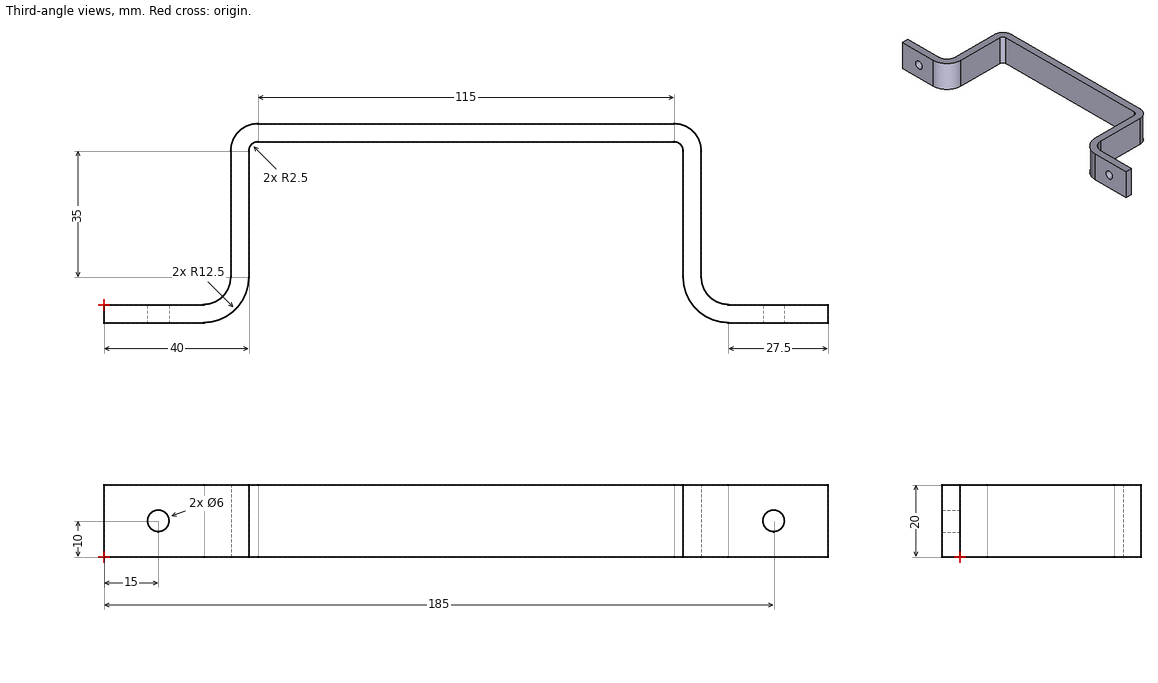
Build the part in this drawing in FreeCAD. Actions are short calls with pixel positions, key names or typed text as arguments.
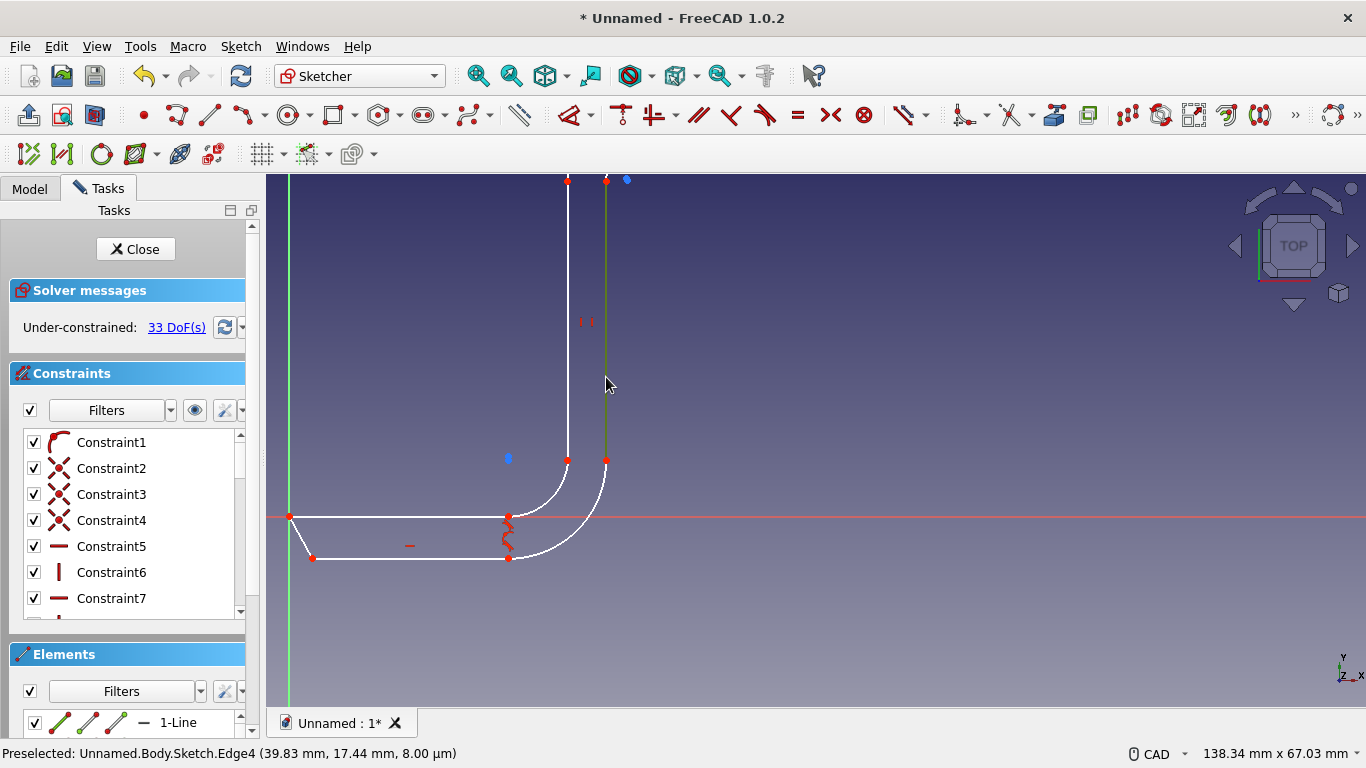
click(553, 548)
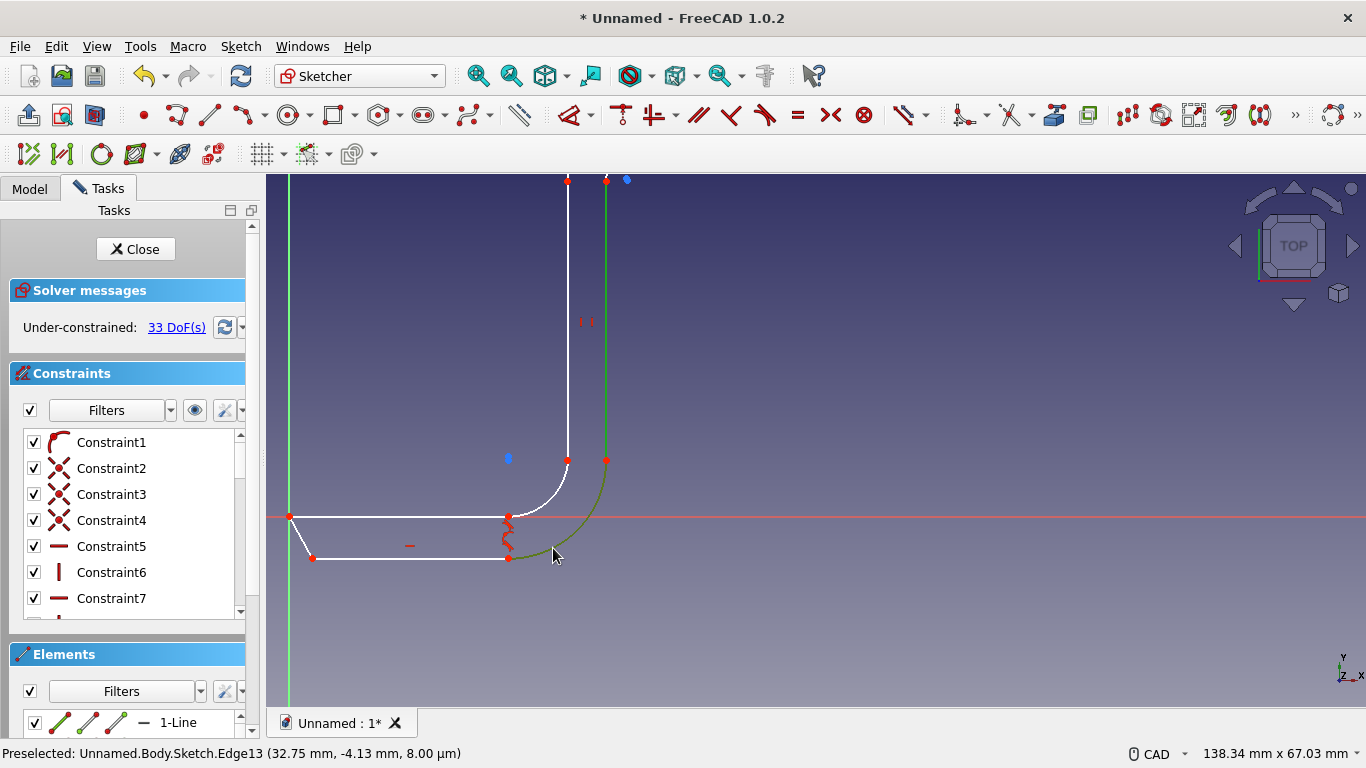
click(765, 116)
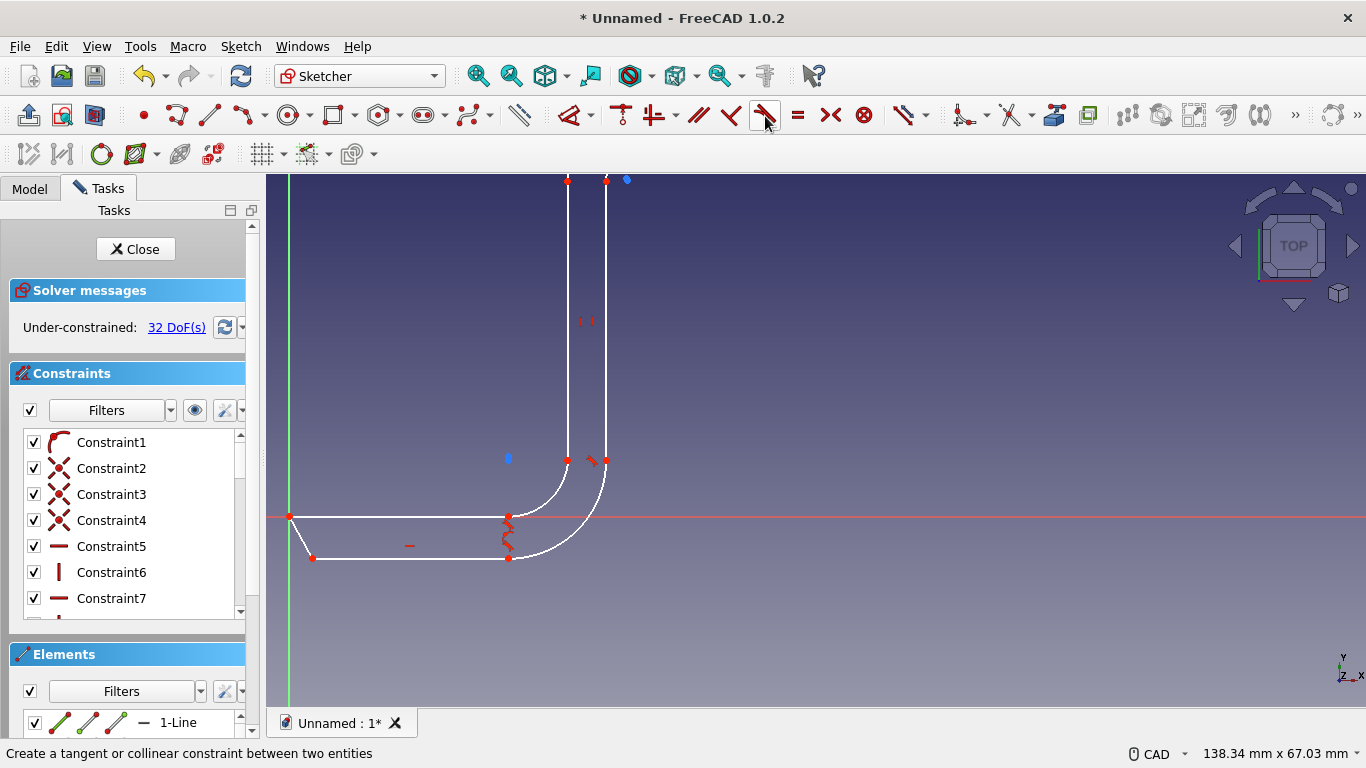
click(606, 377)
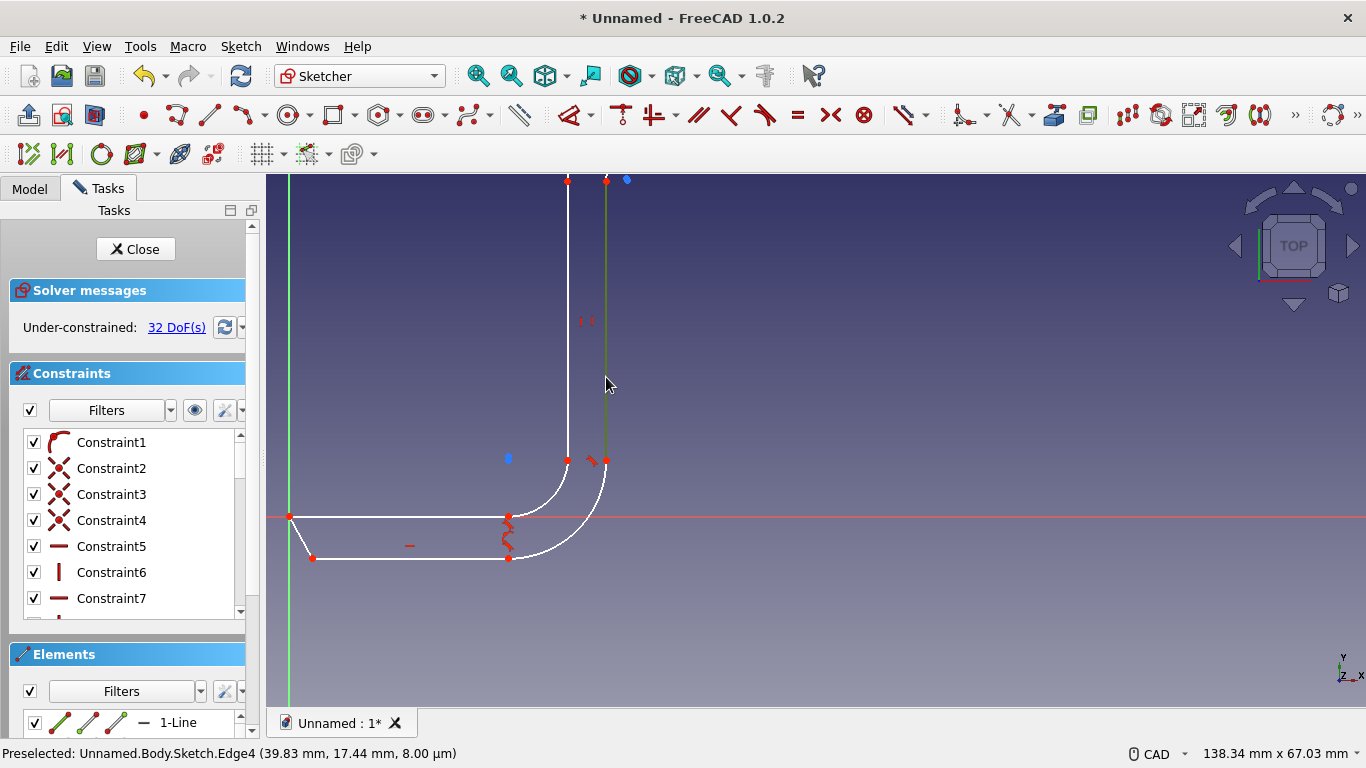
scroll(551, 500, down, 5)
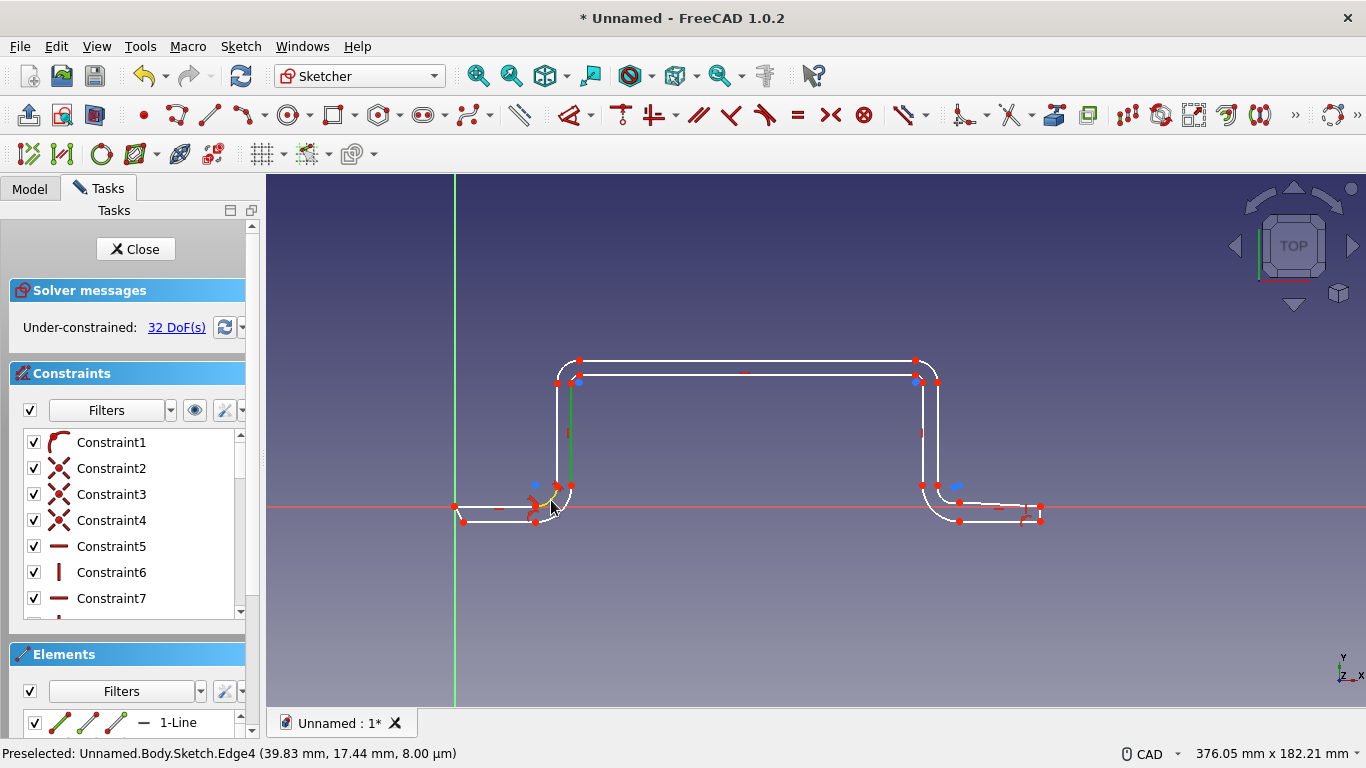
scroll(576, 376, up, 7)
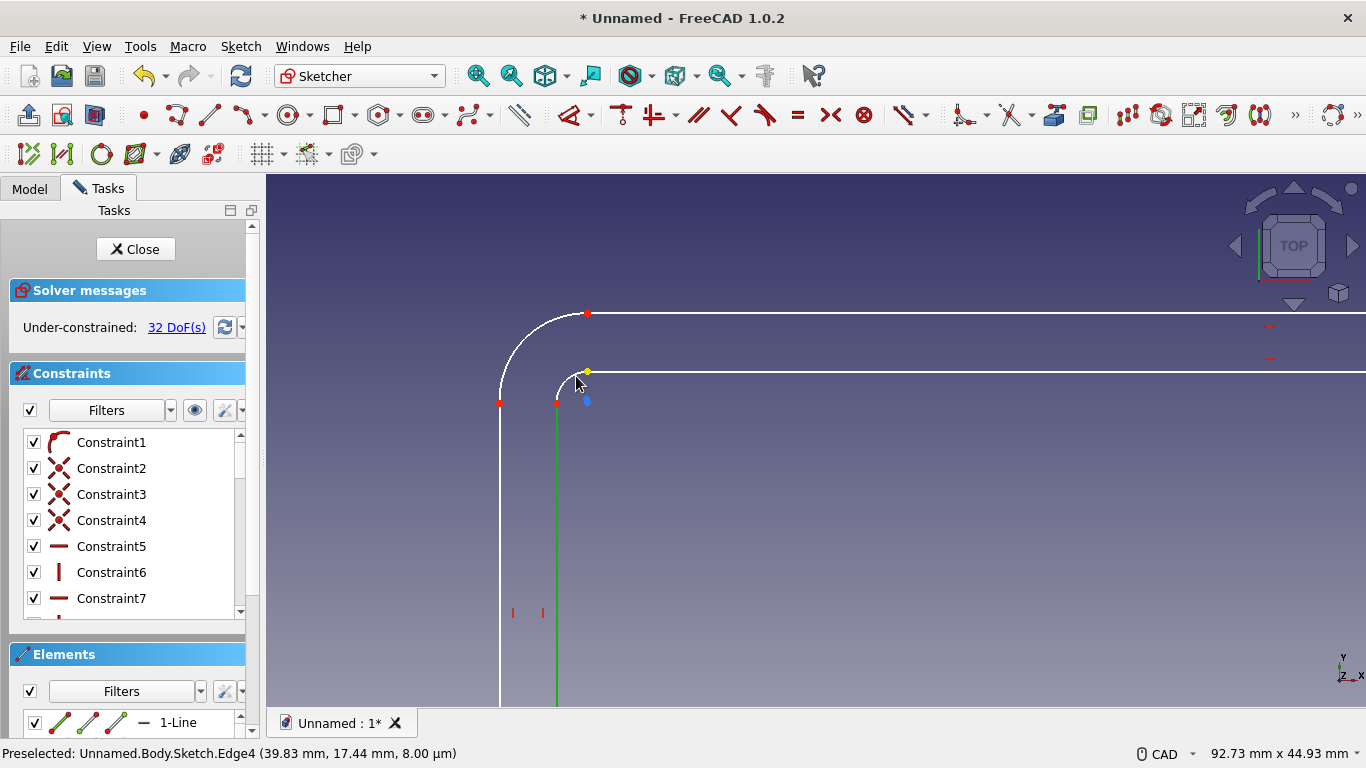
click(573, 375)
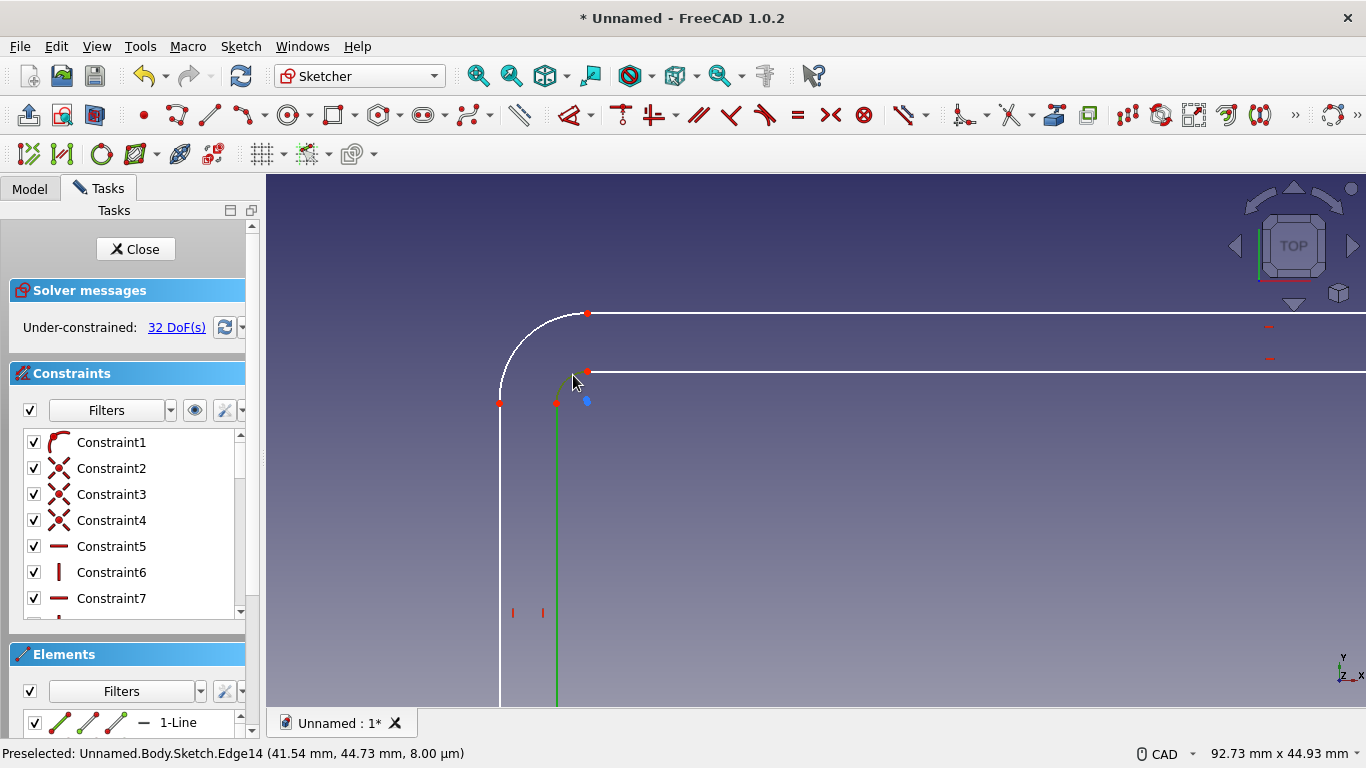
click(765, 116)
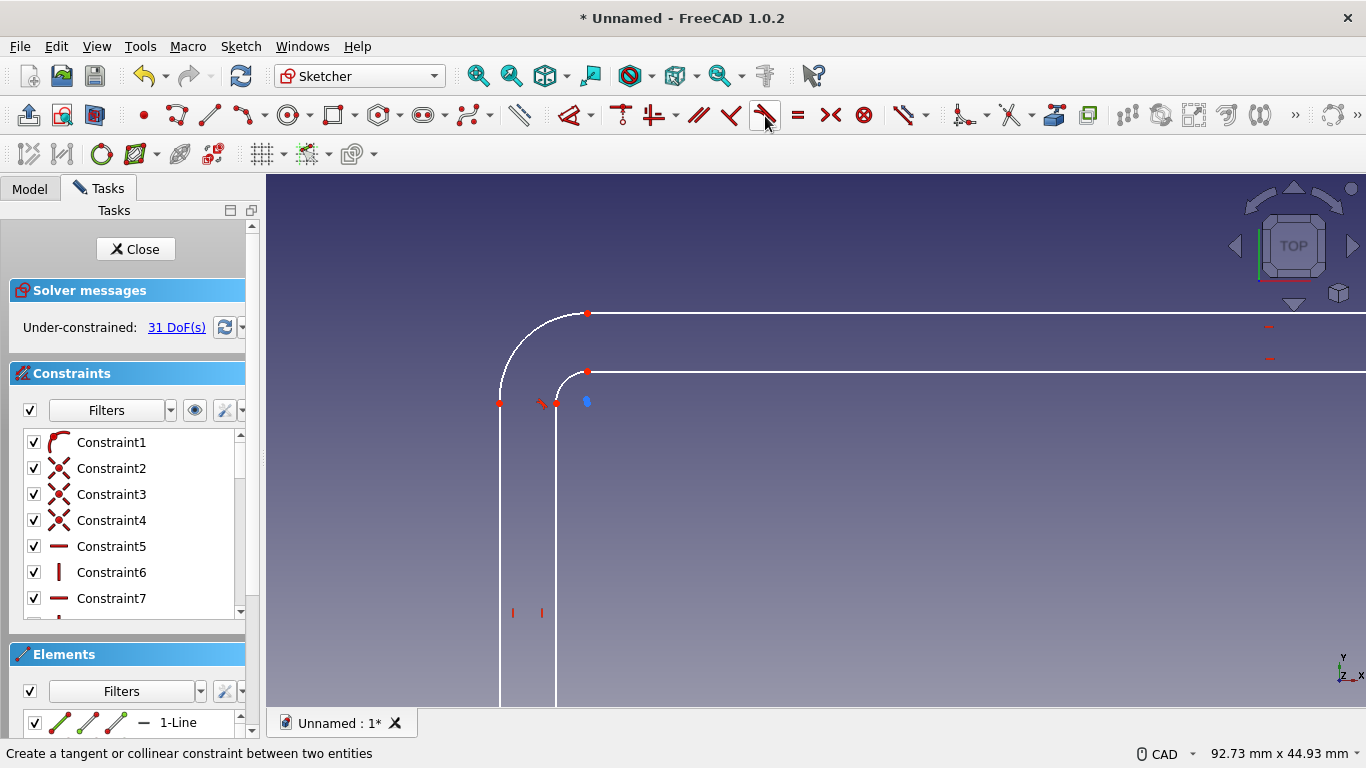
scroll(576, 376, down, 7)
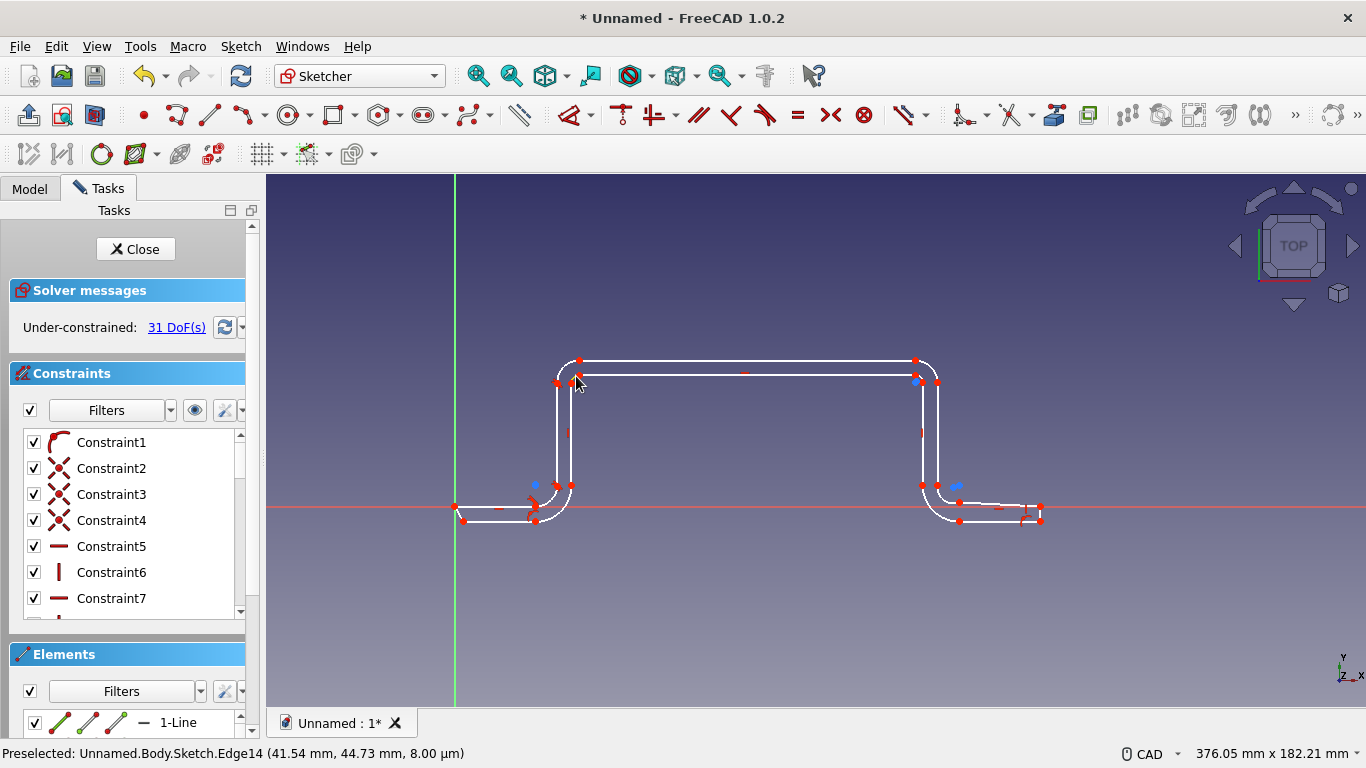
click(680, 375)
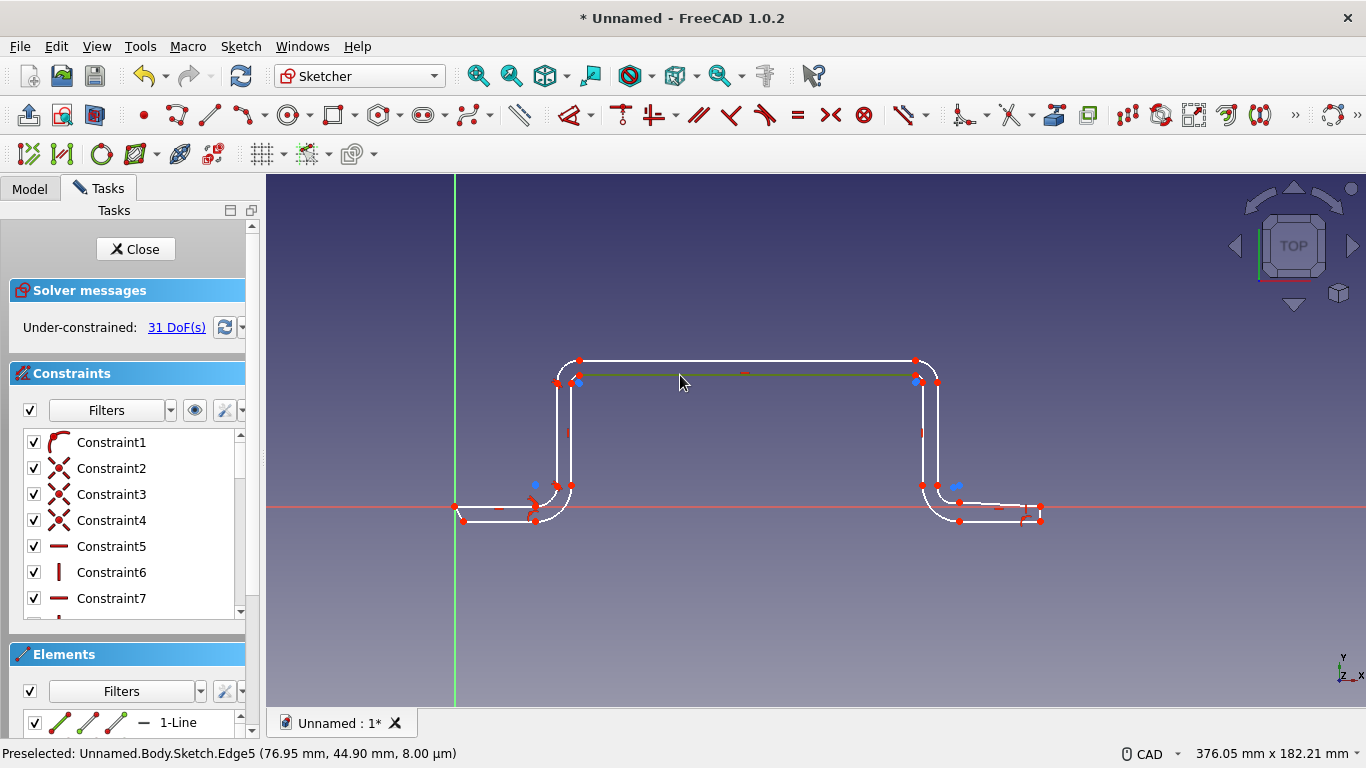
scroll(574, 378, up, 5)